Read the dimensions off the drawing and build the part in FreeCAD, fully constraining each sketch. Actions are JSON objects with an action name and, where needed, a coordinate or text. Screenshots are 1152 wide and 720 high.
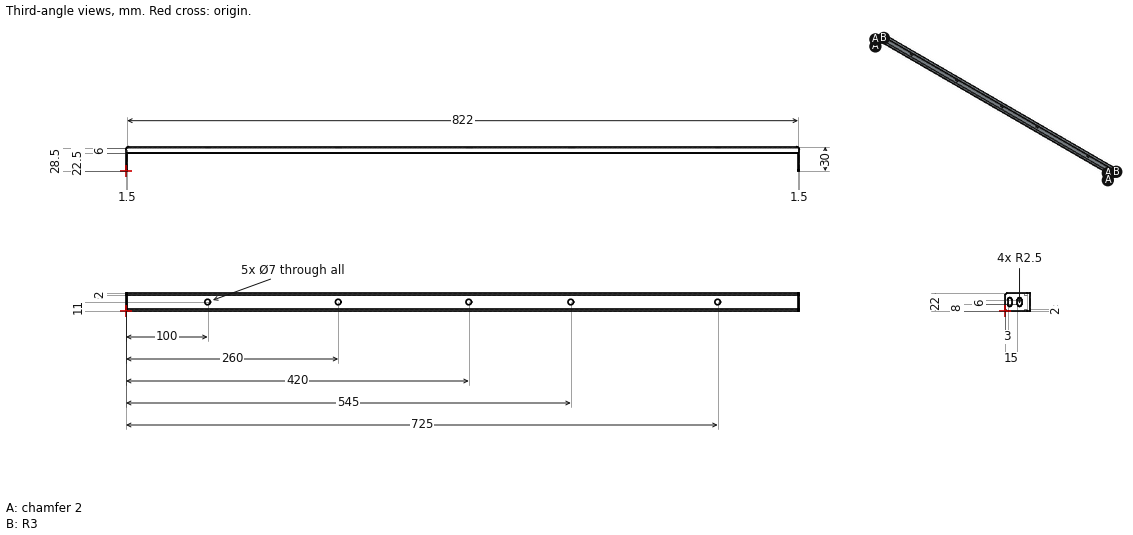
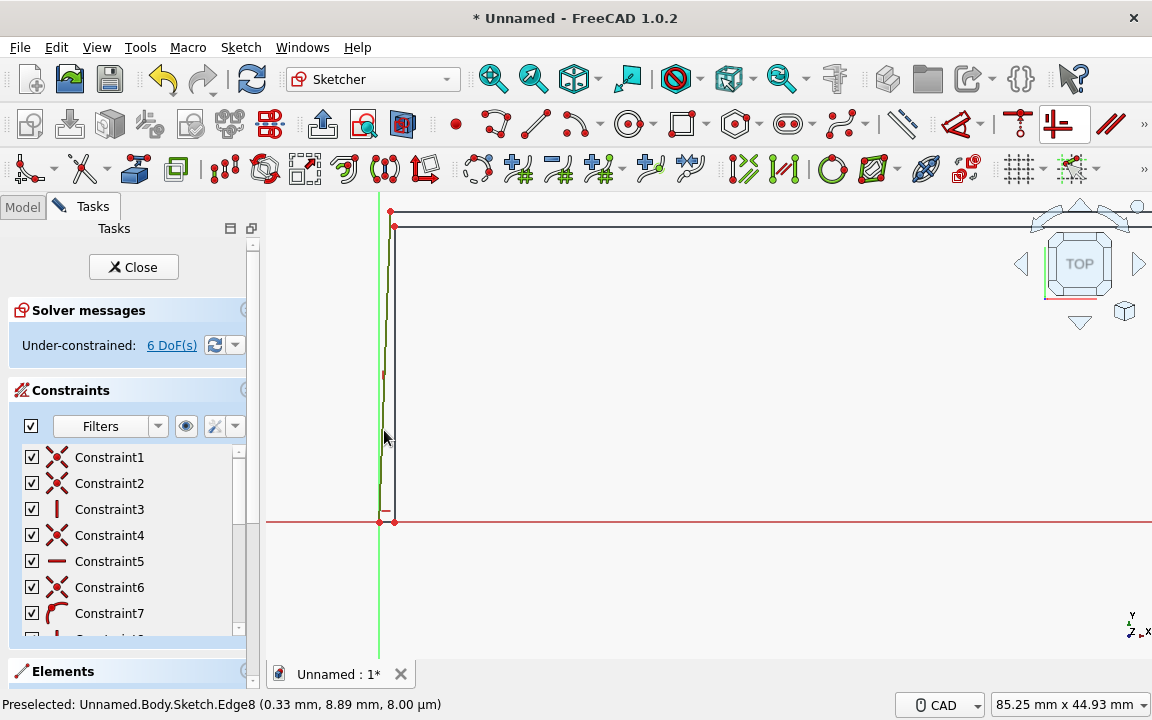
{"action": "key", "text": "v"}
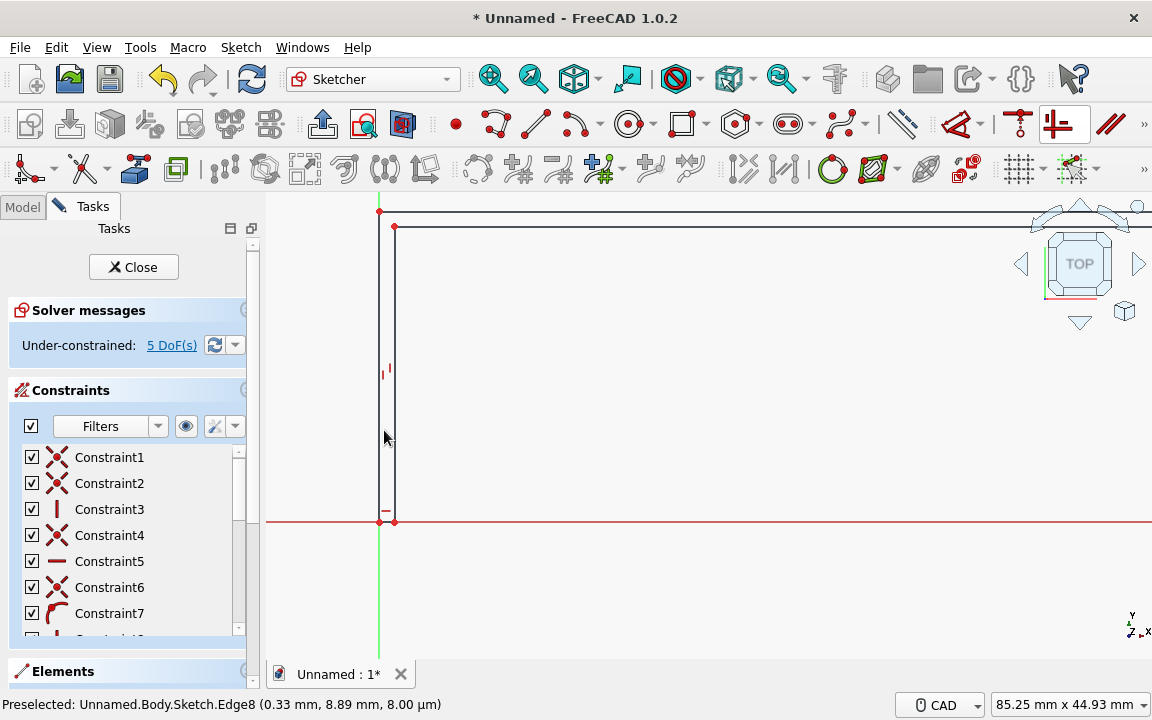
{"action": "scroll", "coordinate": [380, 429], "scroll_direction": "down", "scroll_amount": 14}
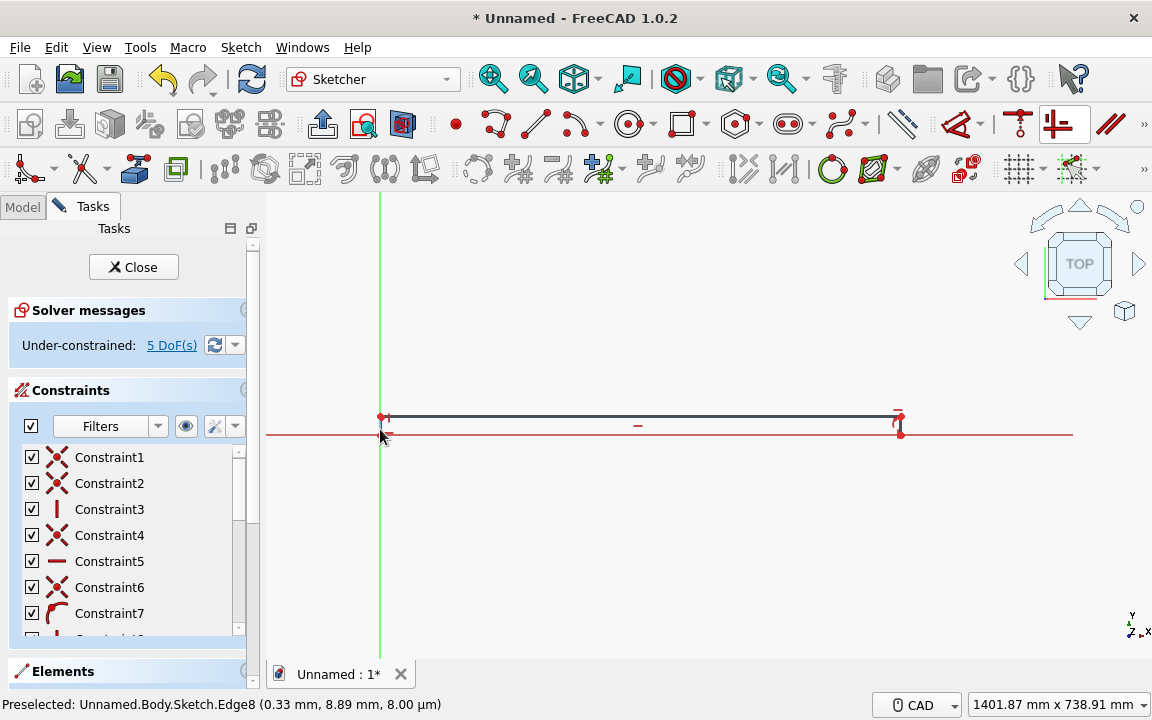
{"action": "scroll", "coordinate": [901, 429], "scroll_direction": "up", "scroll_amount": 13}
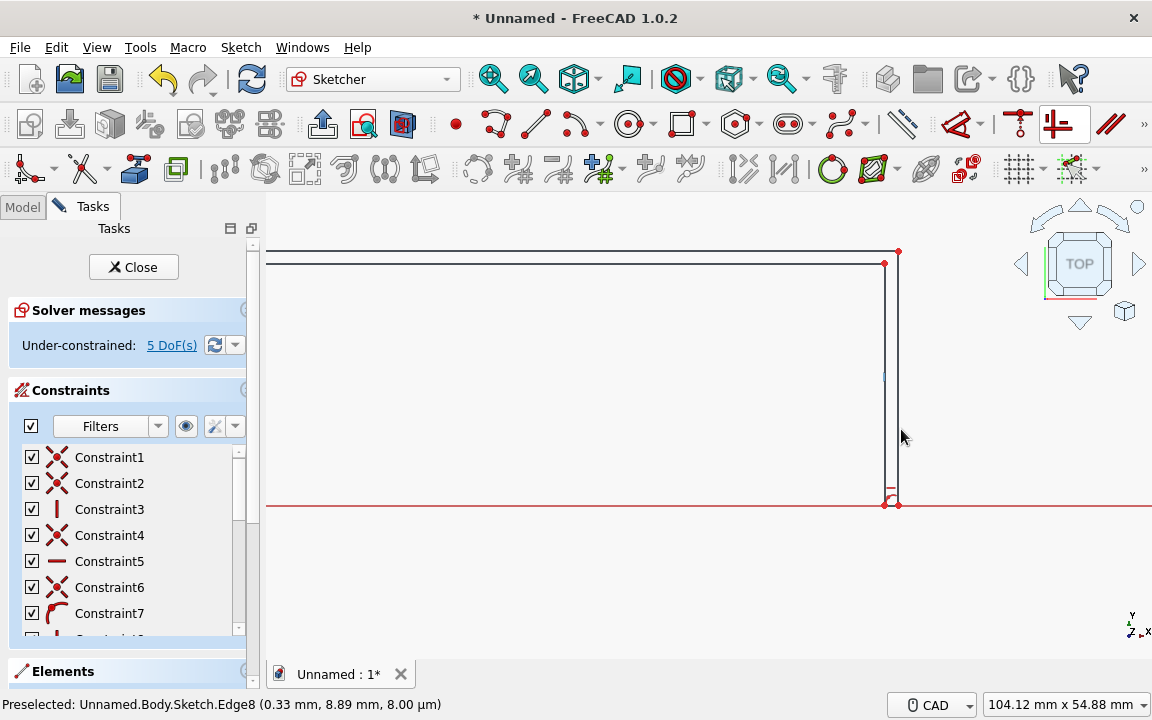
{"action": "left_click", "coordinate": [898, 429]}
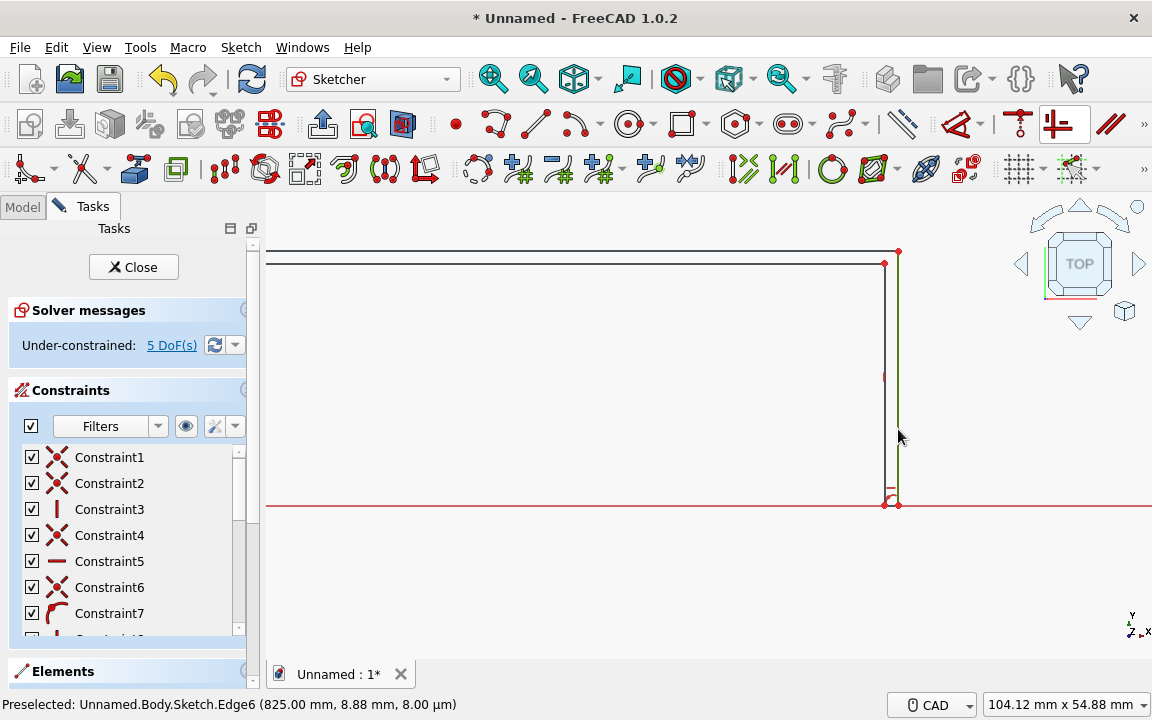
{"action": "left_click", "coordinate": [982, 124]}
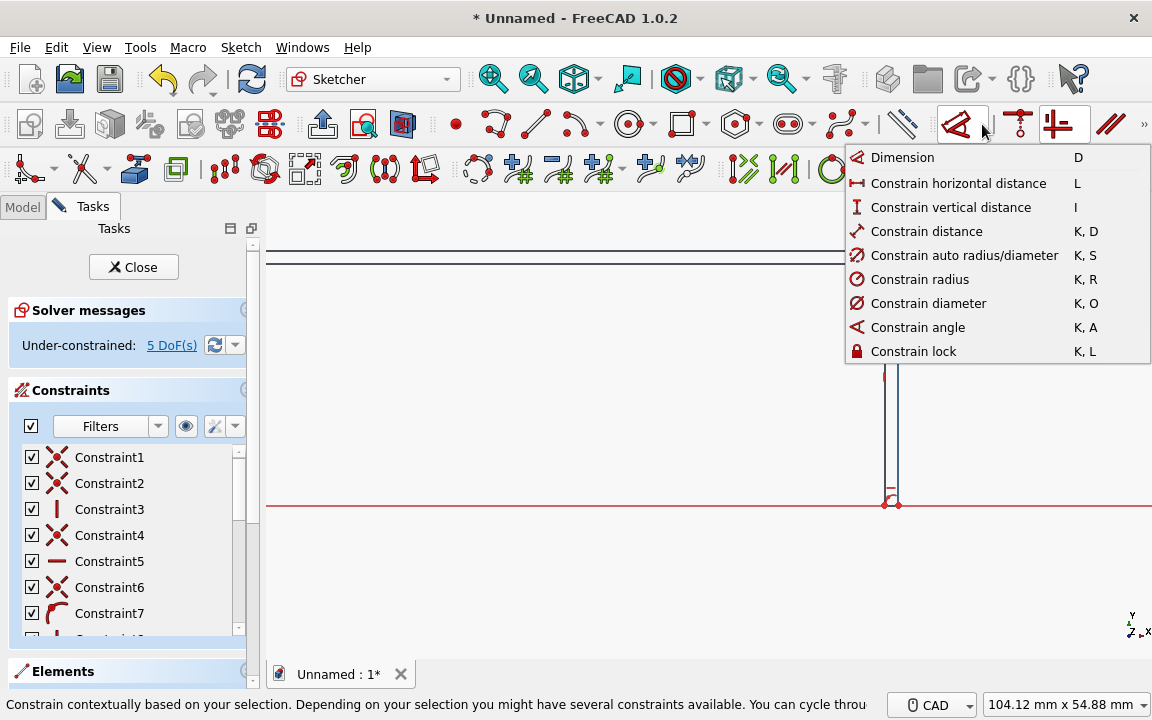
{"action": "left_click", "coordinate": [998, 207]}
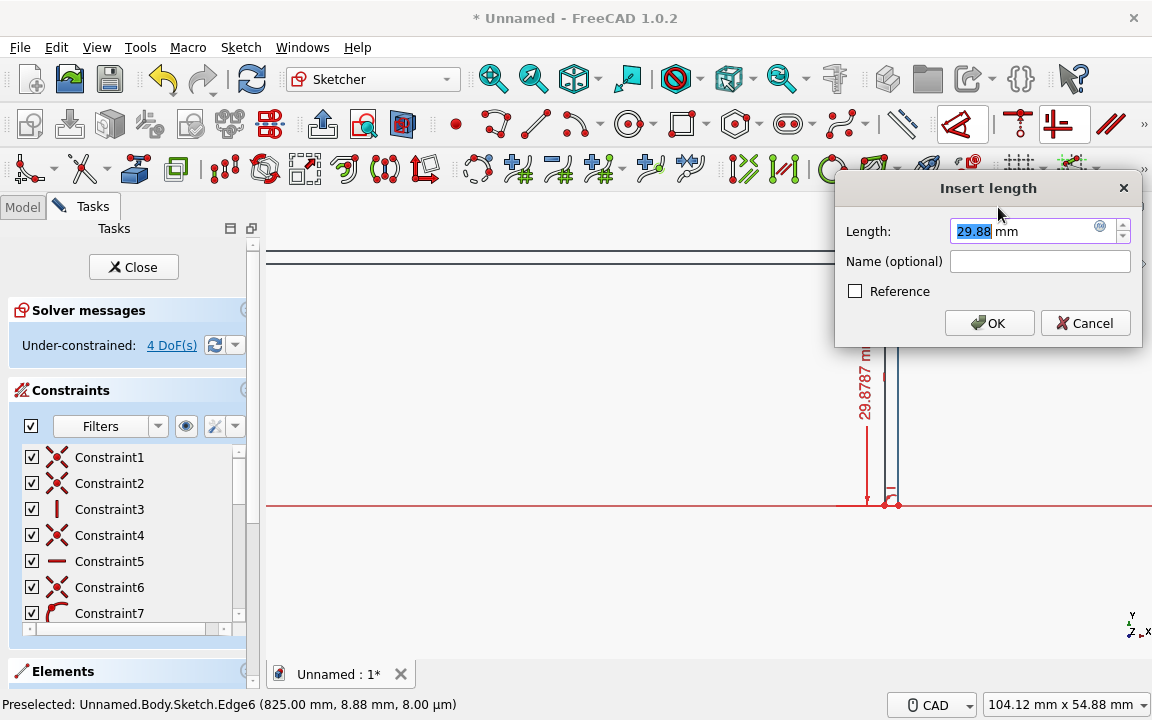
{"action": "type", "text": "30"}
{"action": "key", "text": "Return"}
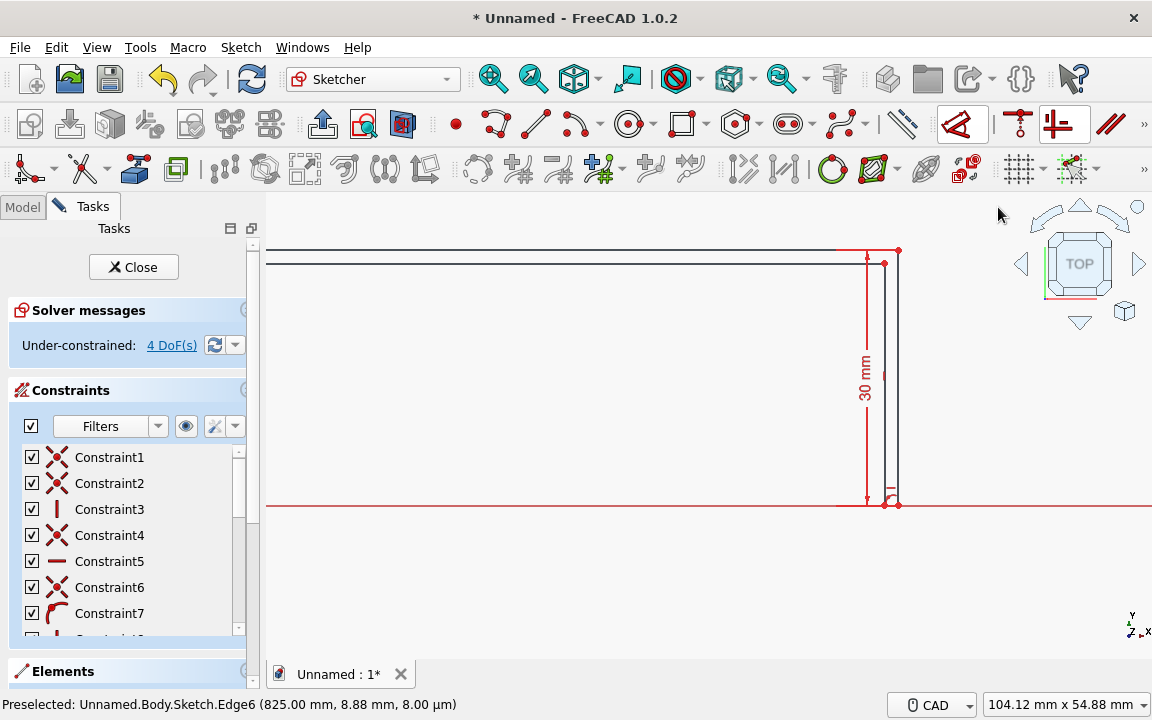
{"action": "scroll", "coordinate": [901, 429], "scroll_direction": "down", "scroll_amount": 13}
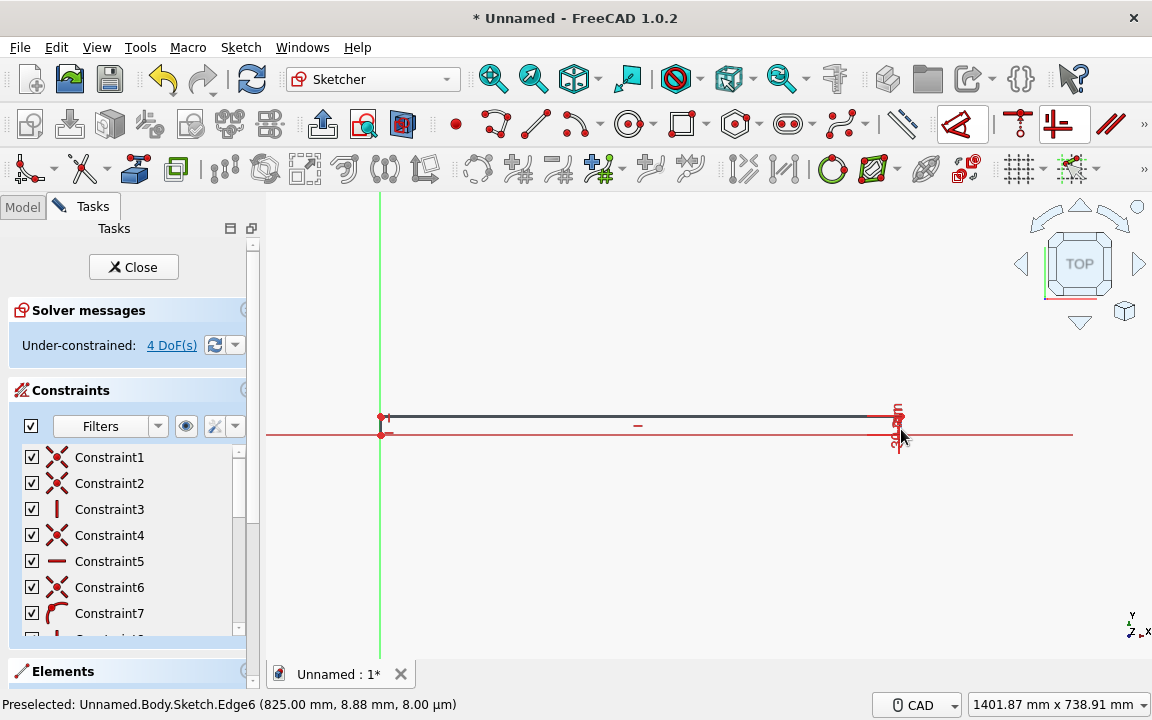
{"action": "scroll", "coordinate": [381, 435], "scroll_direction": "up", "scroll_amount": 19}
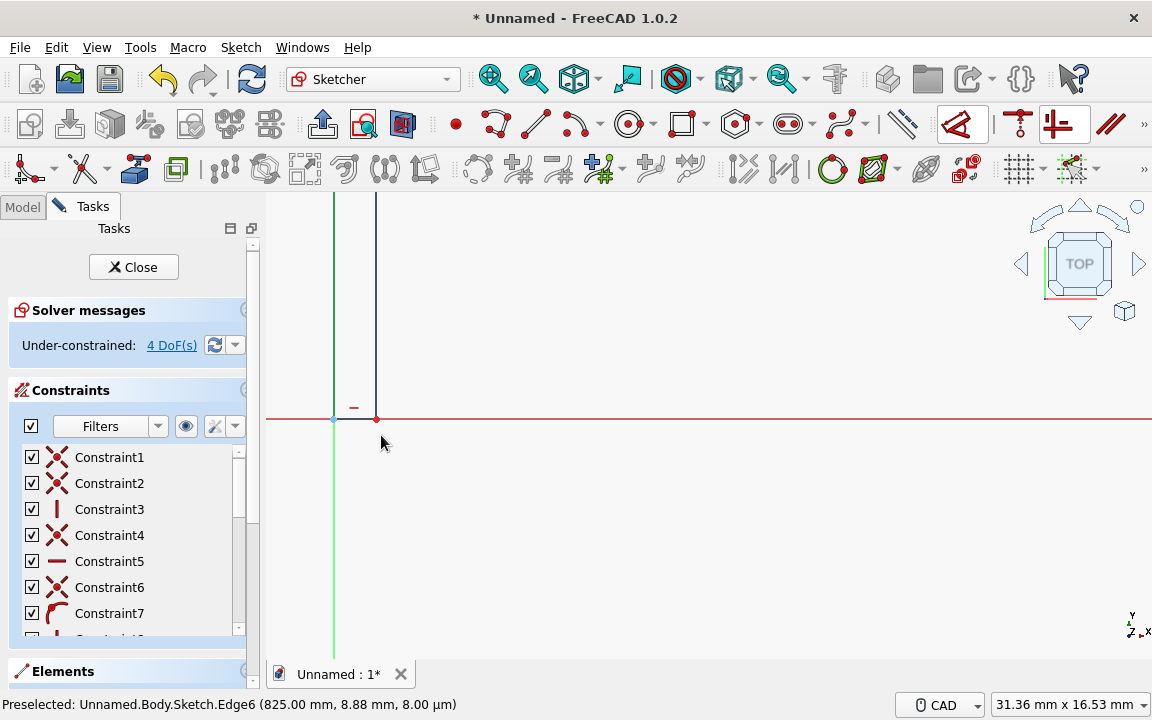
{"action": "left_click", "coordinate": [355, 419]}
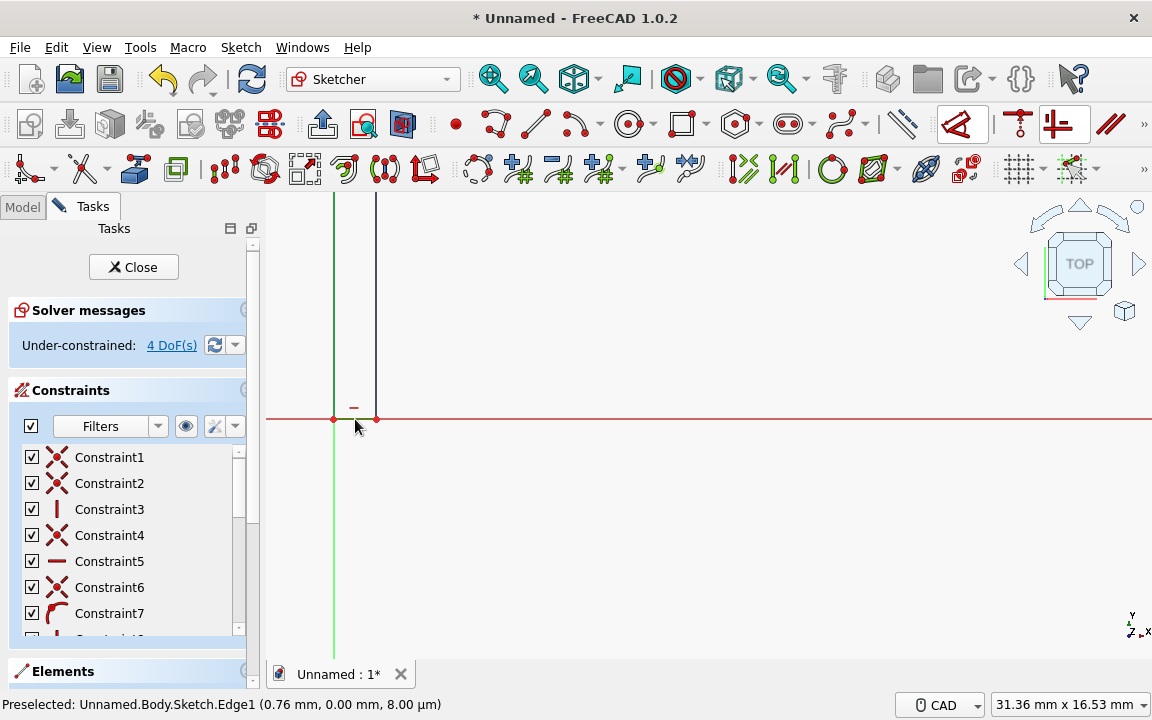
{"action": "key", "text": "l"}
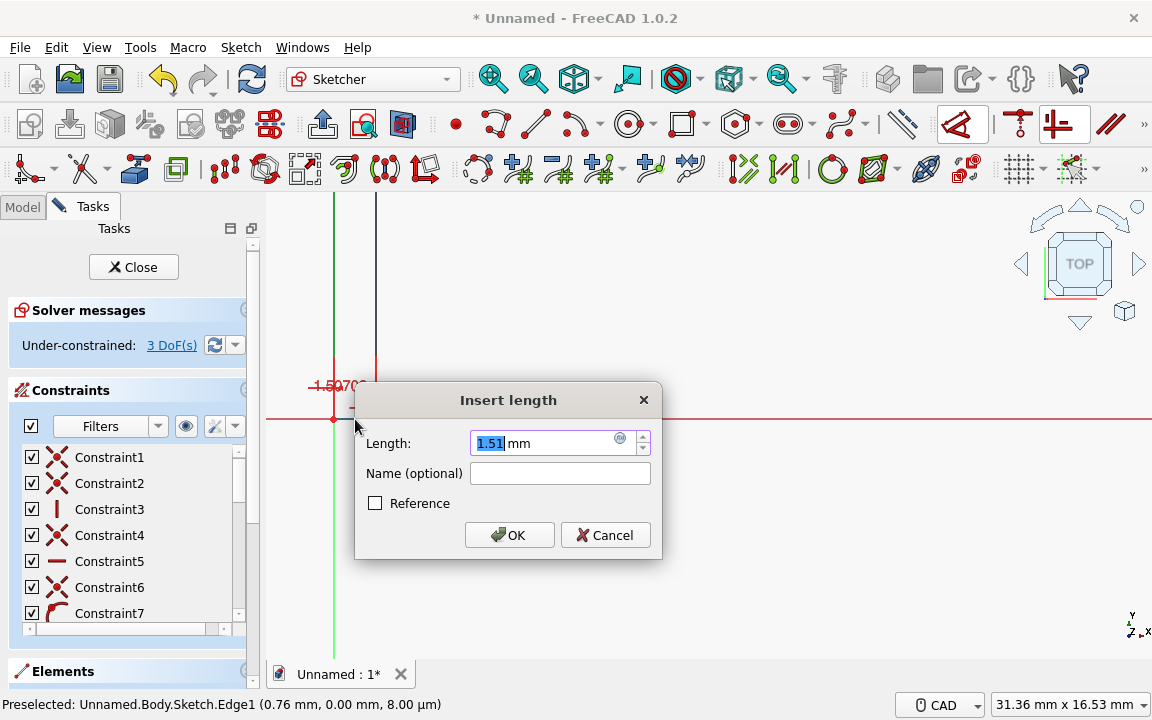
{"action": "type", "text": "1.5"}
{"action": "key", "text": "Return"}